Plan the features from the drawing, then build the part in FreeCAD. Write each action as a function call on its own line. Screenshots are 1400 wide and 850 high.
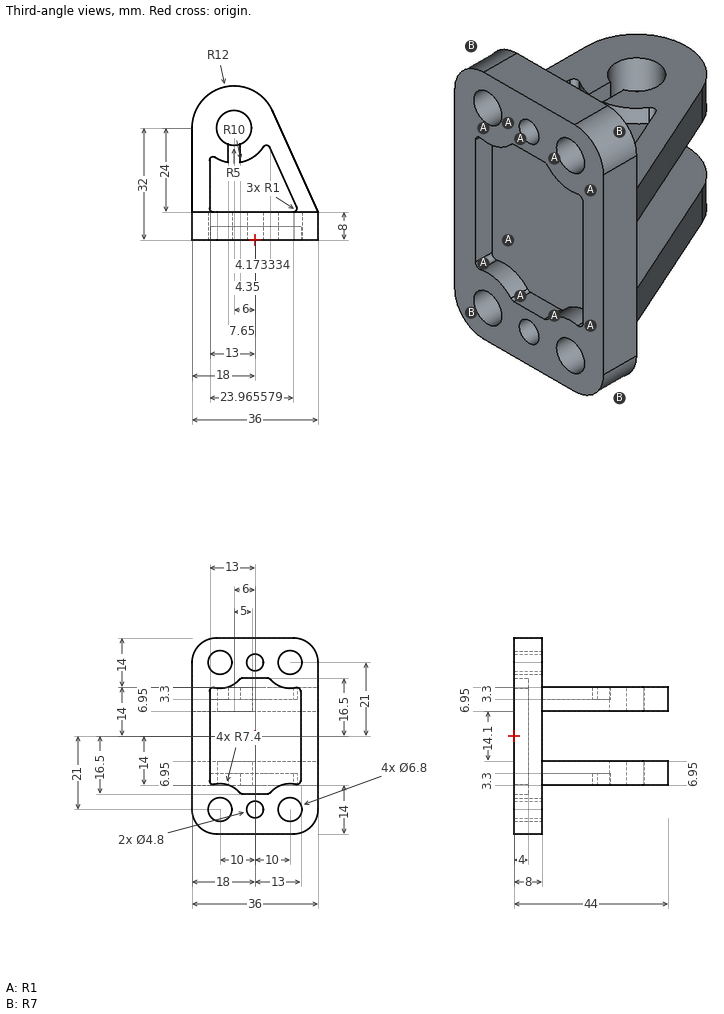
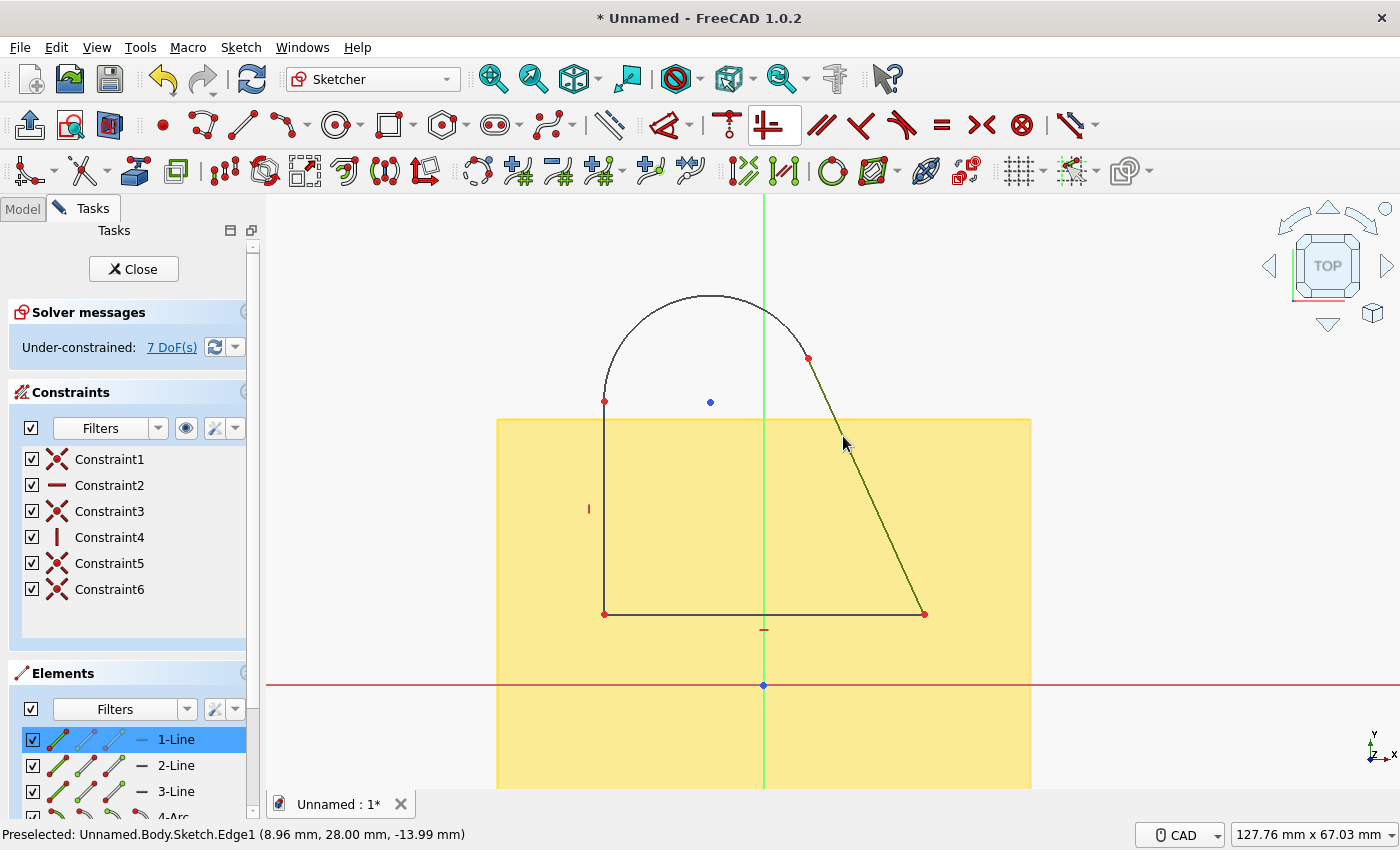
click(746, 302)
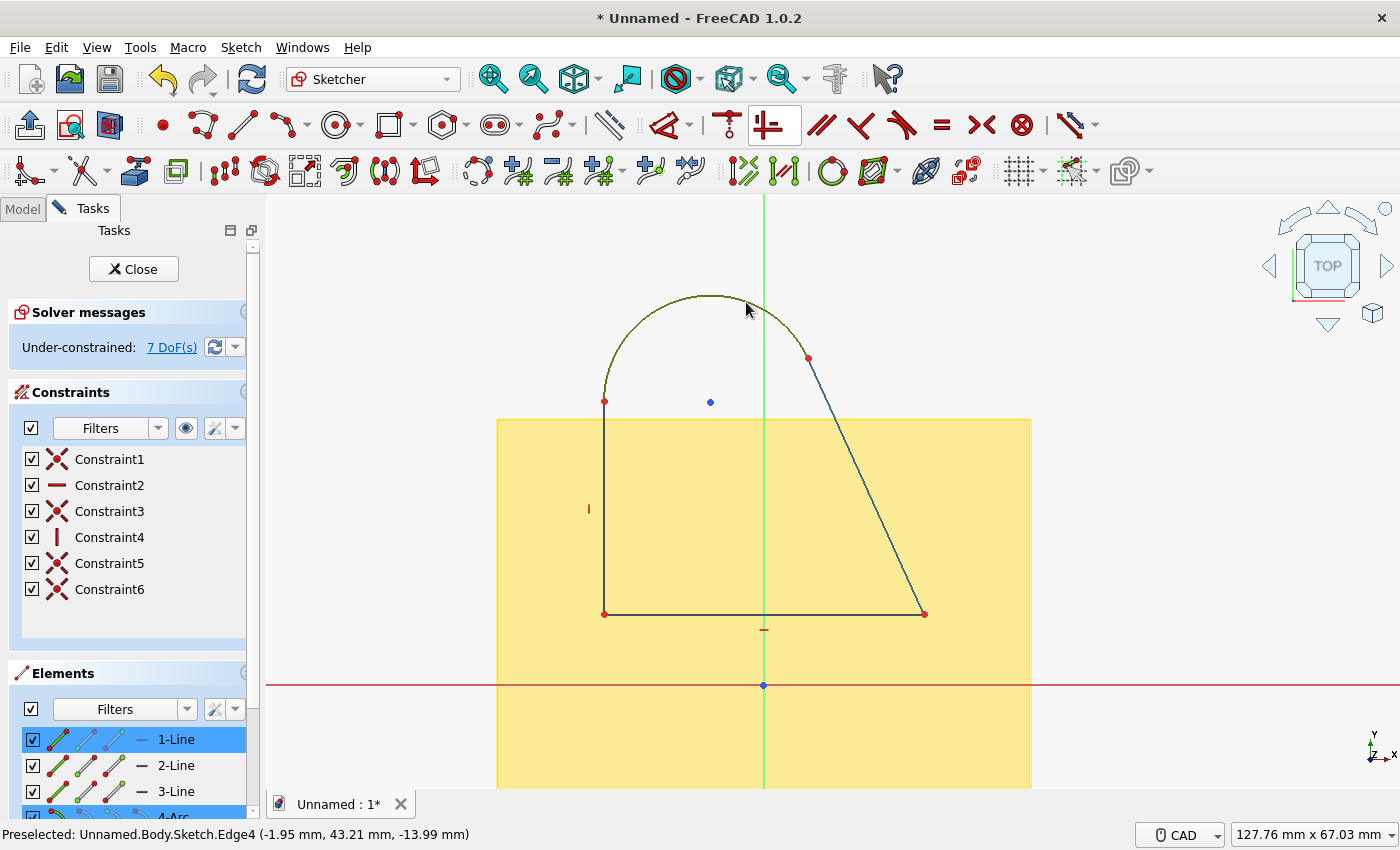
key(t)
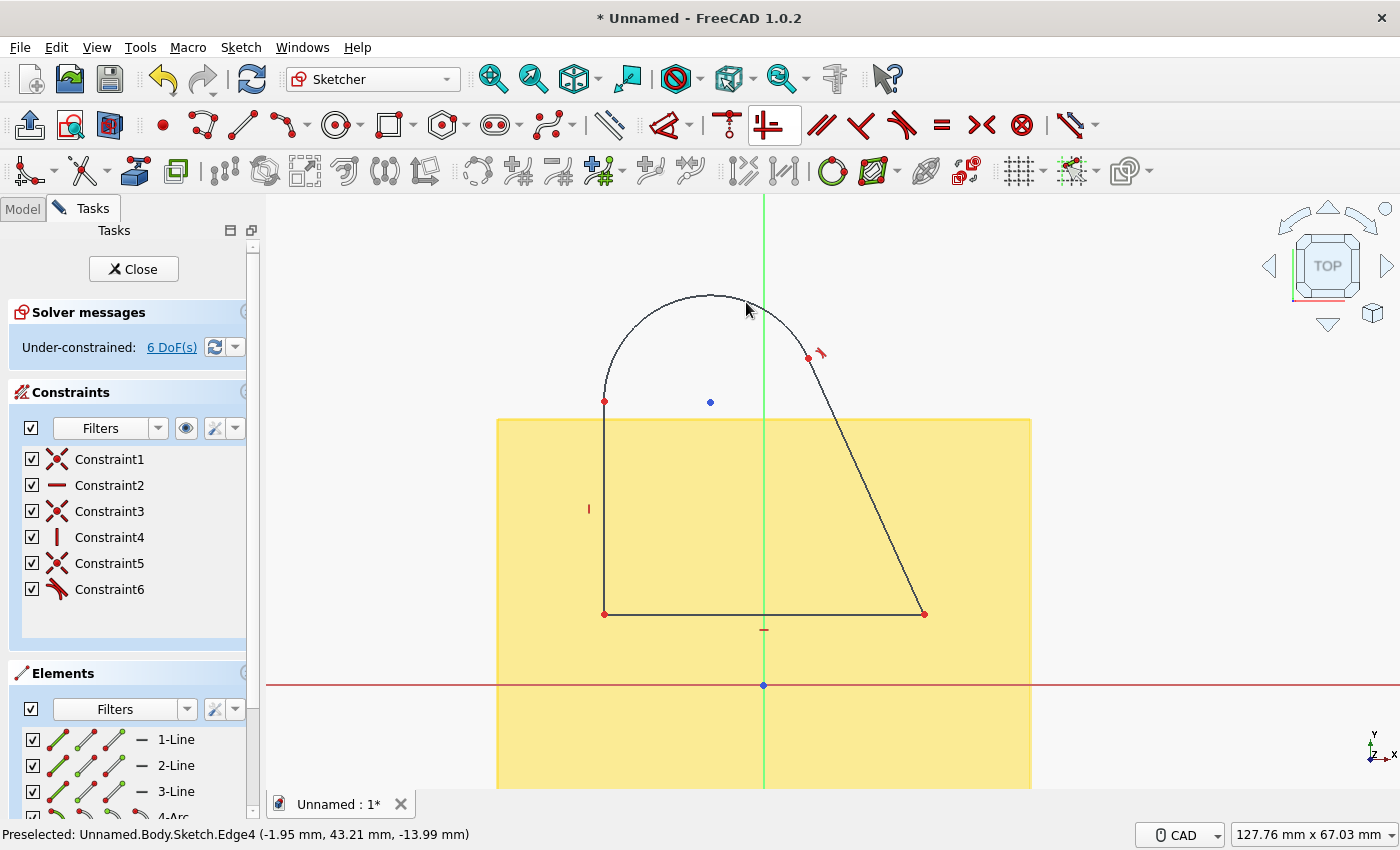
click(604, 551)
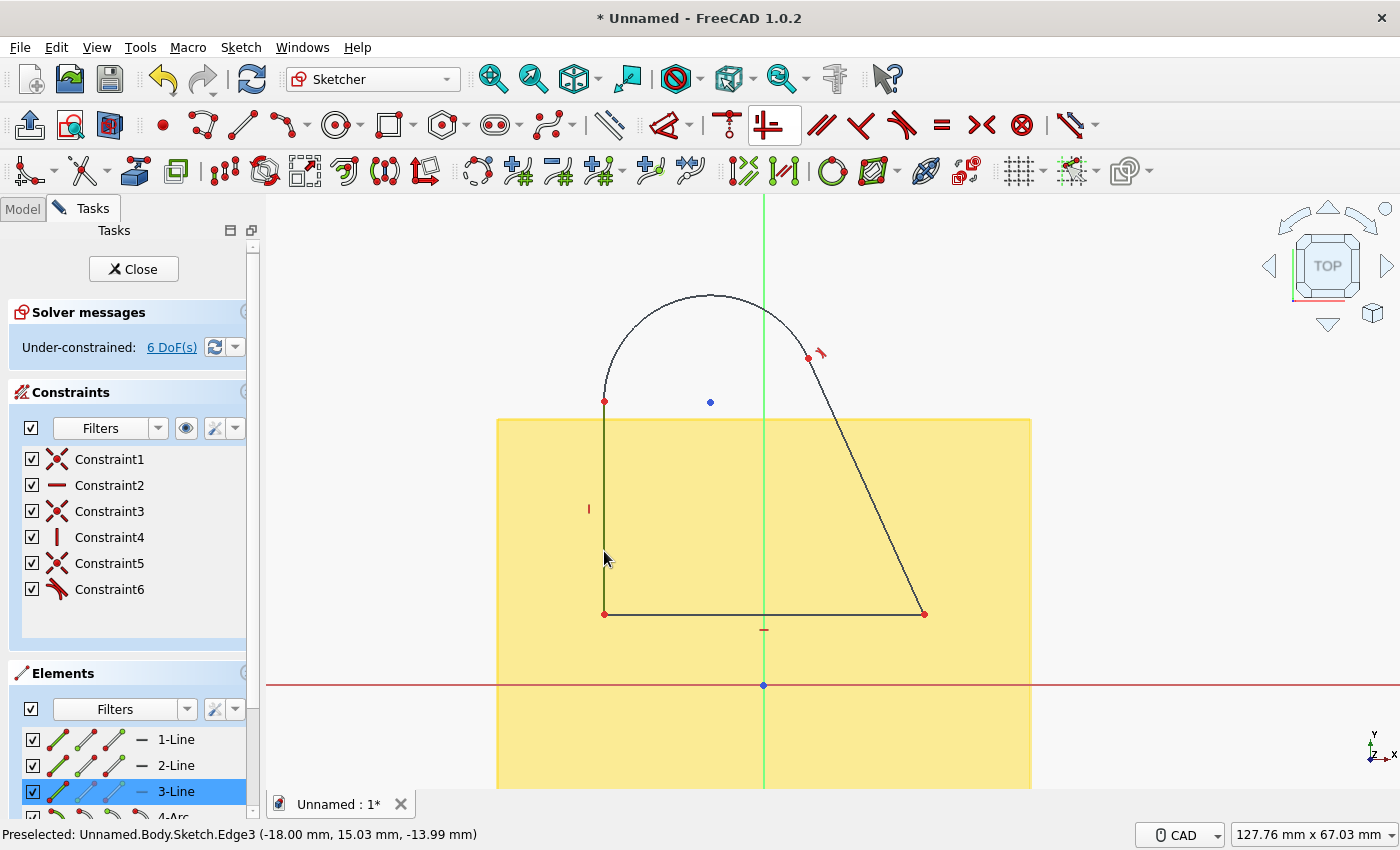
click(745, 301)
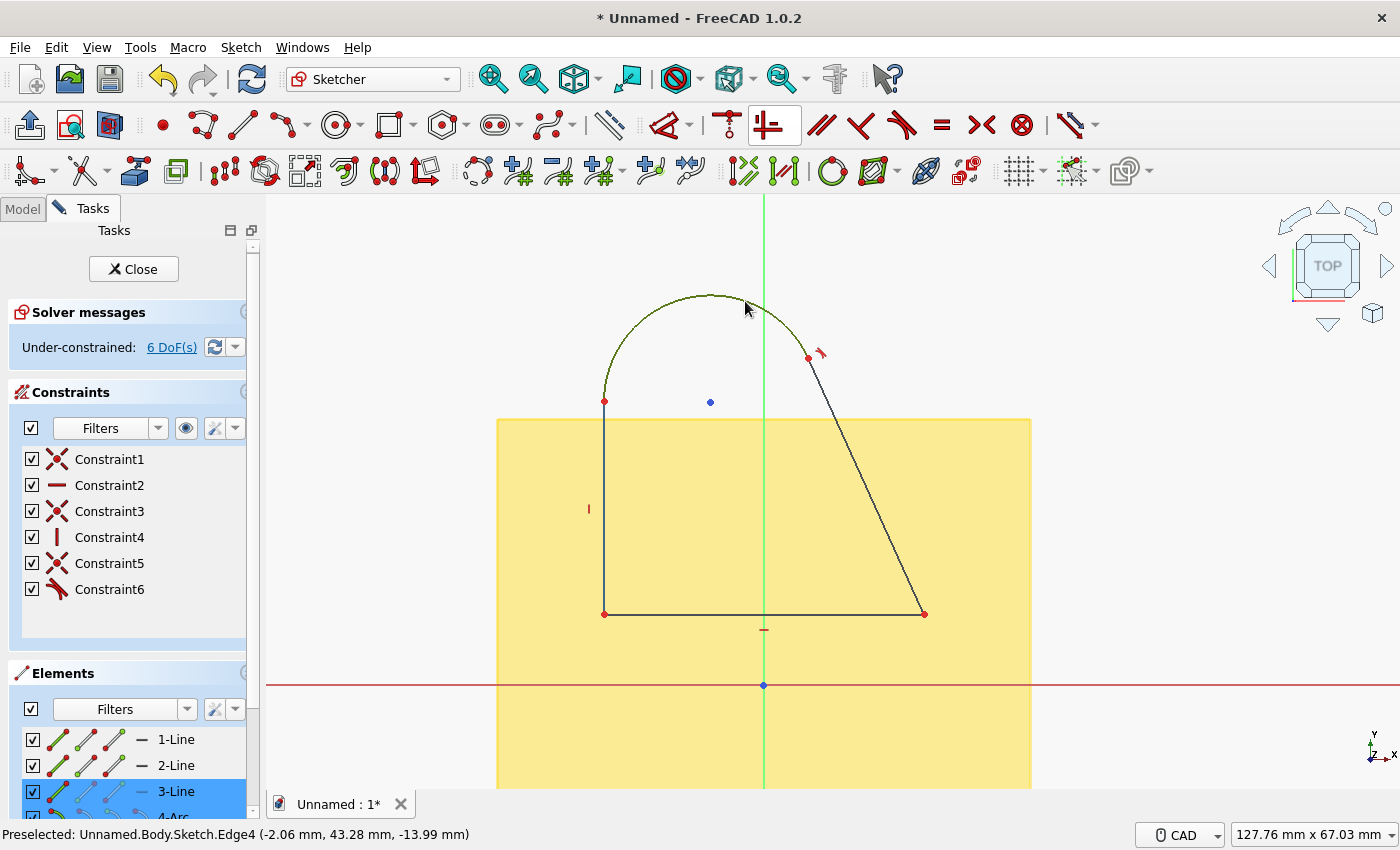
key(t)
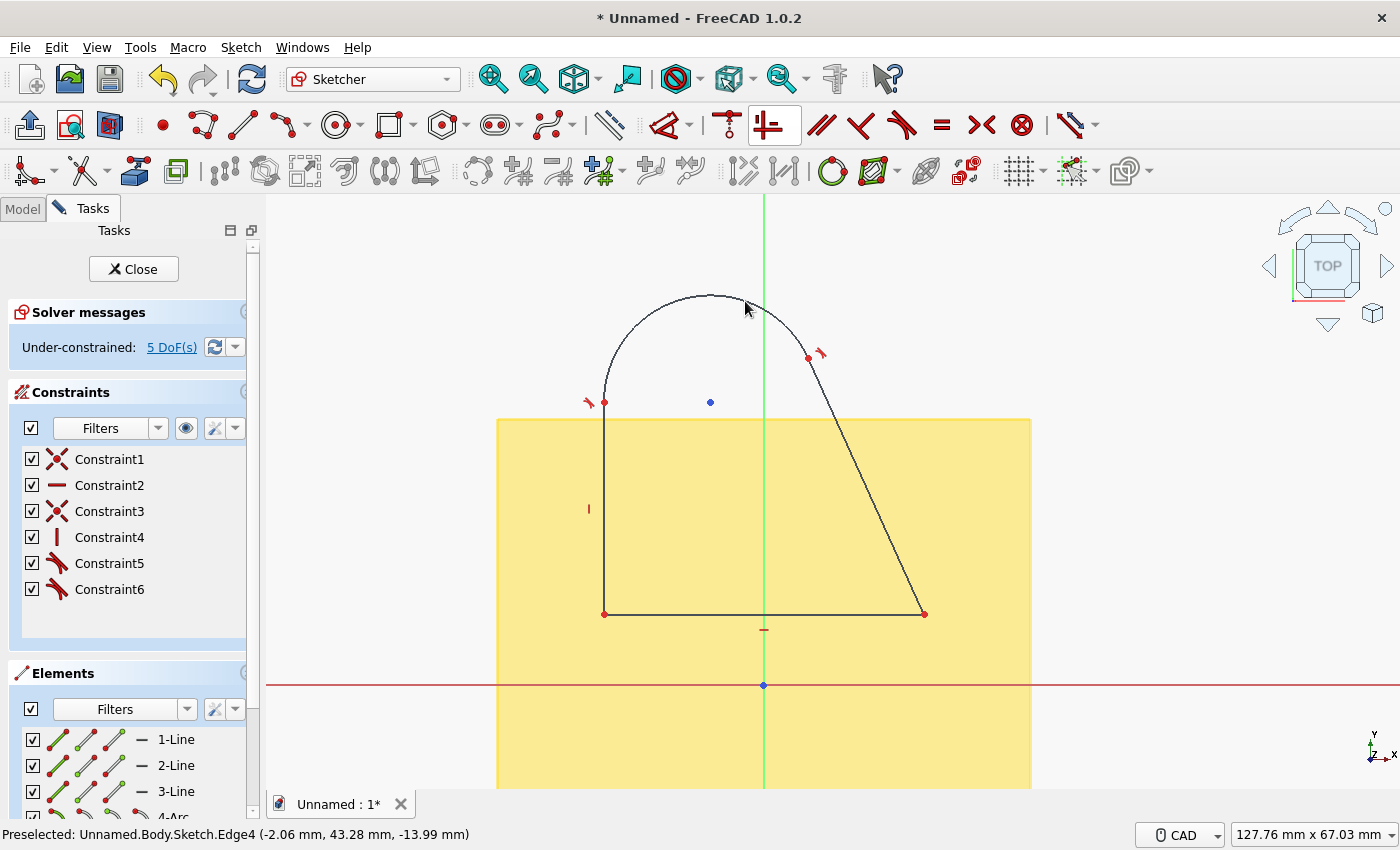
click(745, 301)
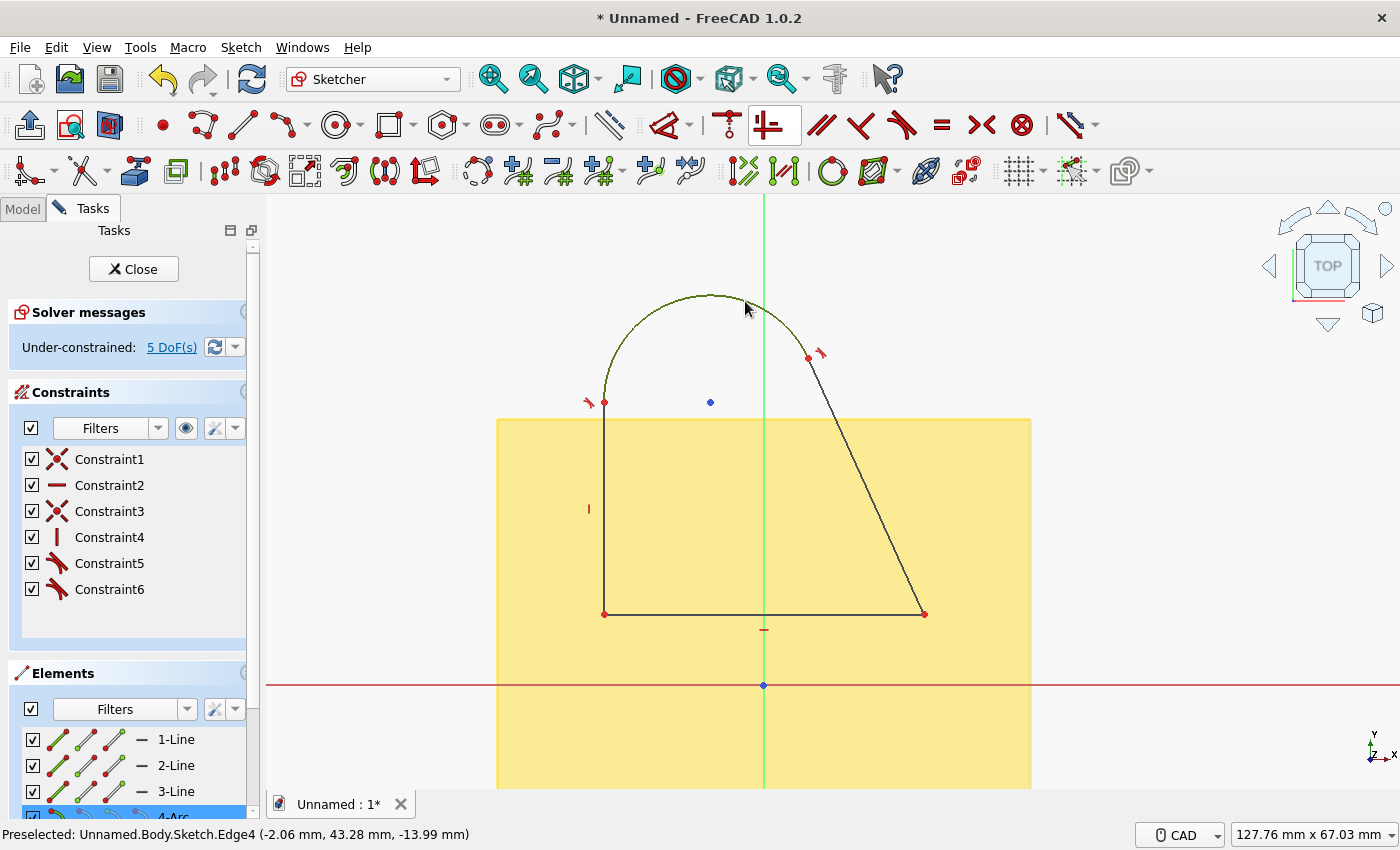
key(k)
key(r)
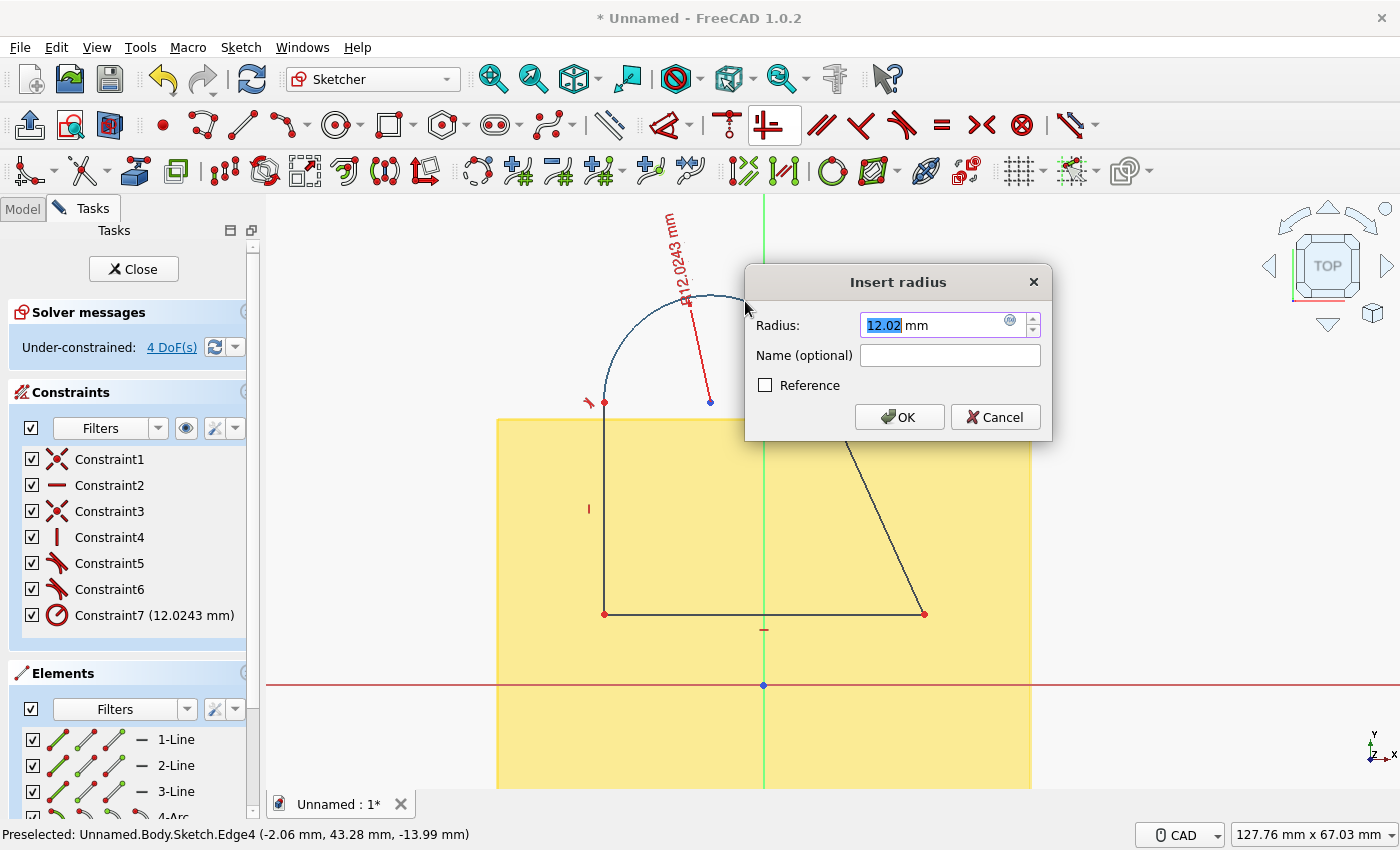
text(12)
key(Return)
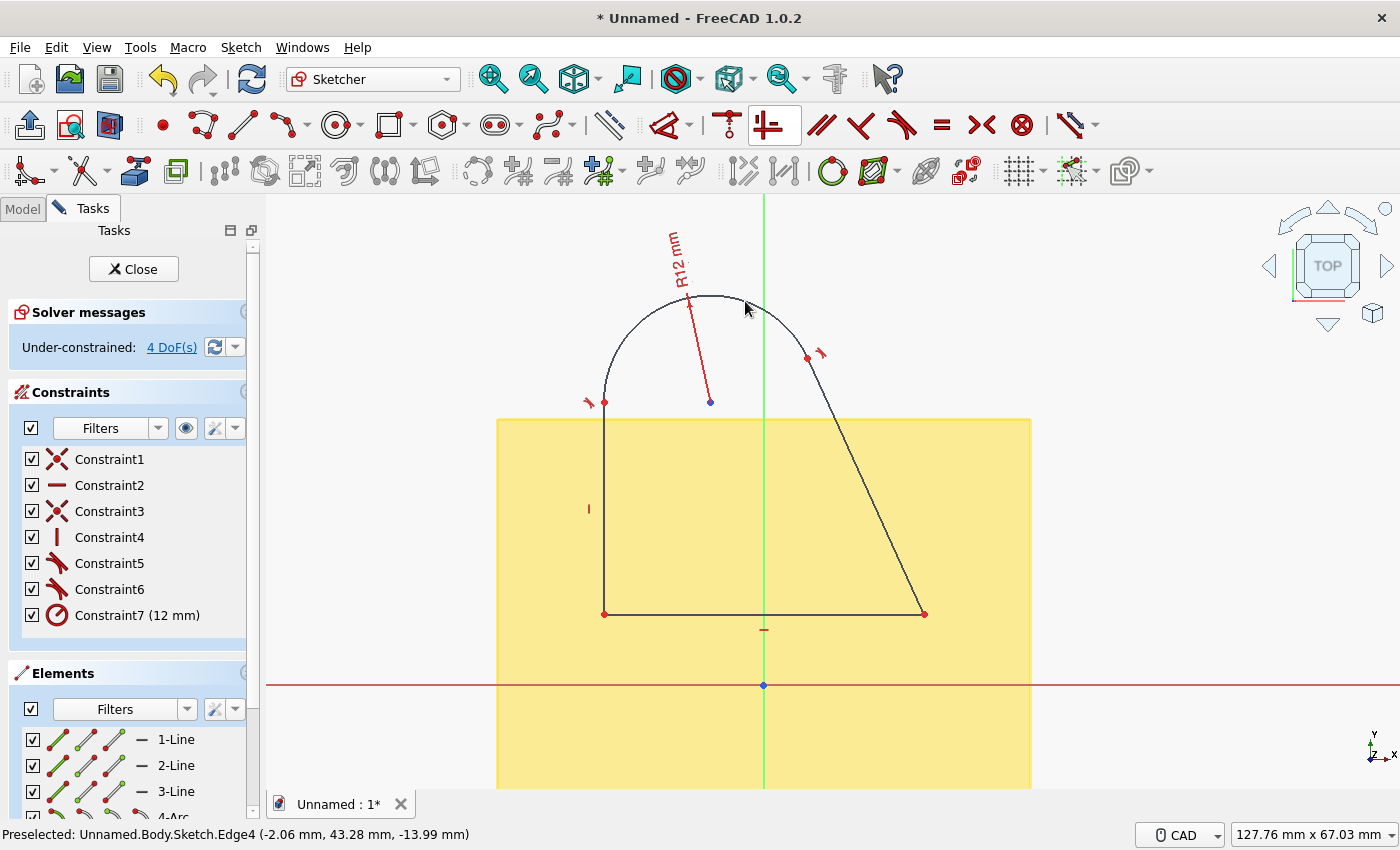
click(828, 615)